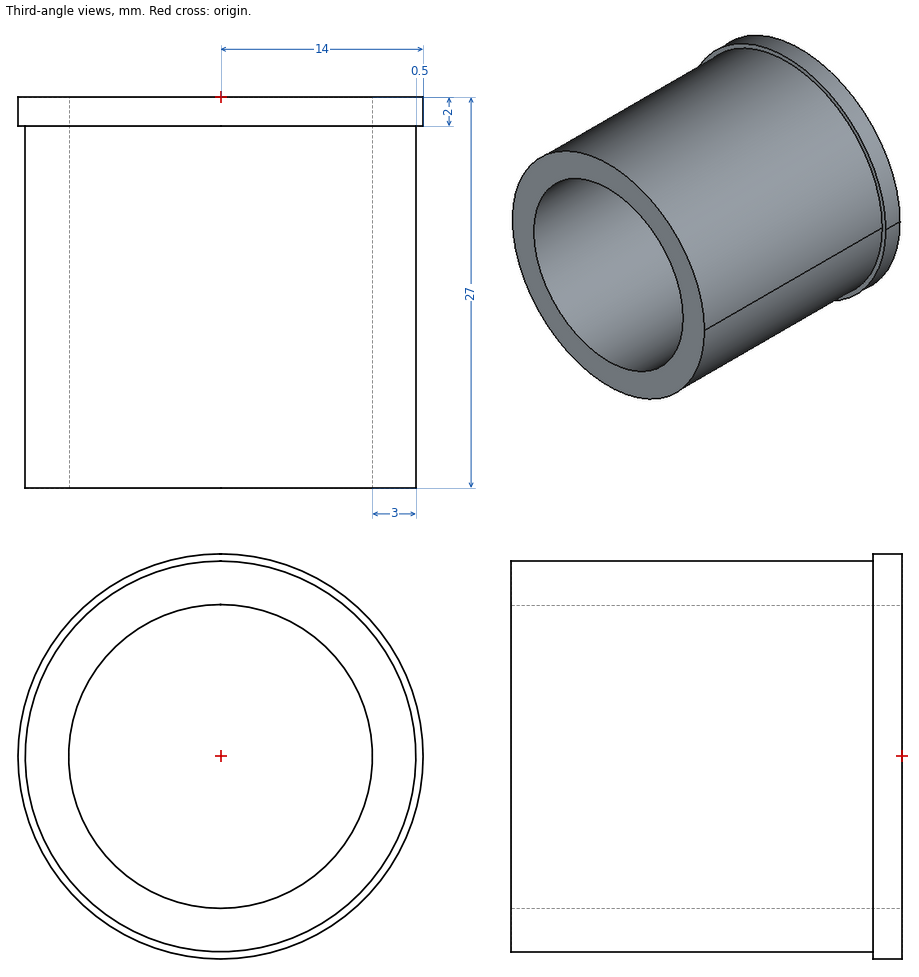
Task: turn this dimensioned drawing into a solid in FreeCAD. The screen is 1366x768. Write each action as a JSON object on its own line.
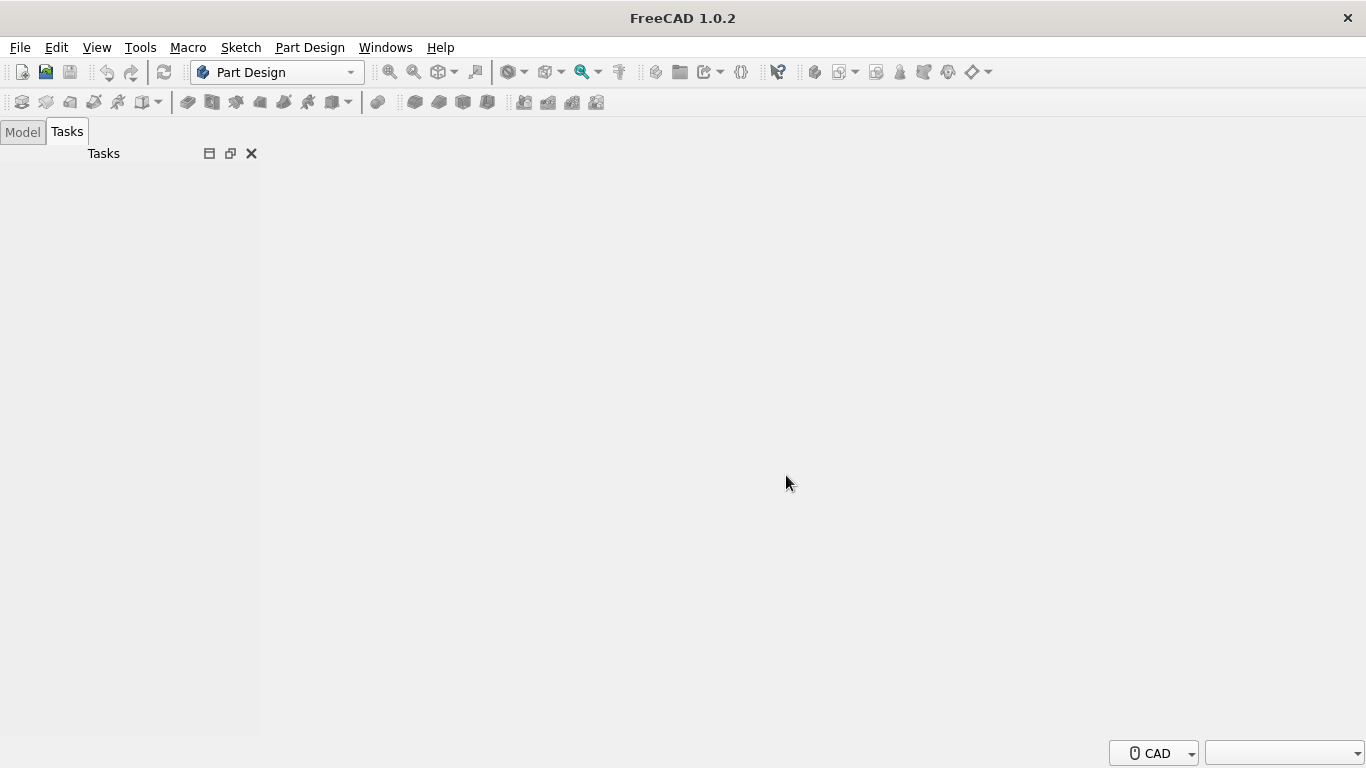
{"action": "key", "text": "ctrl+n"}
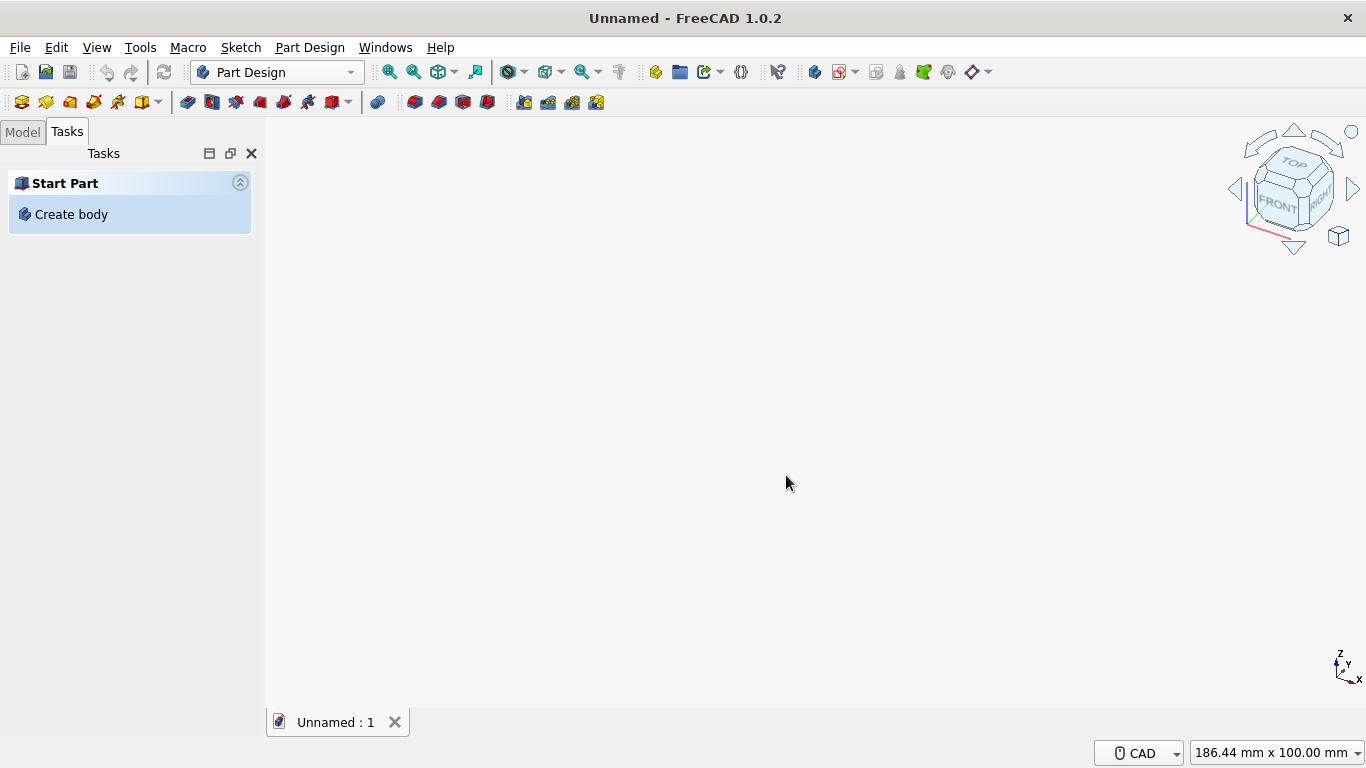
{"action": "left_click", "coordinate": [840, 72]}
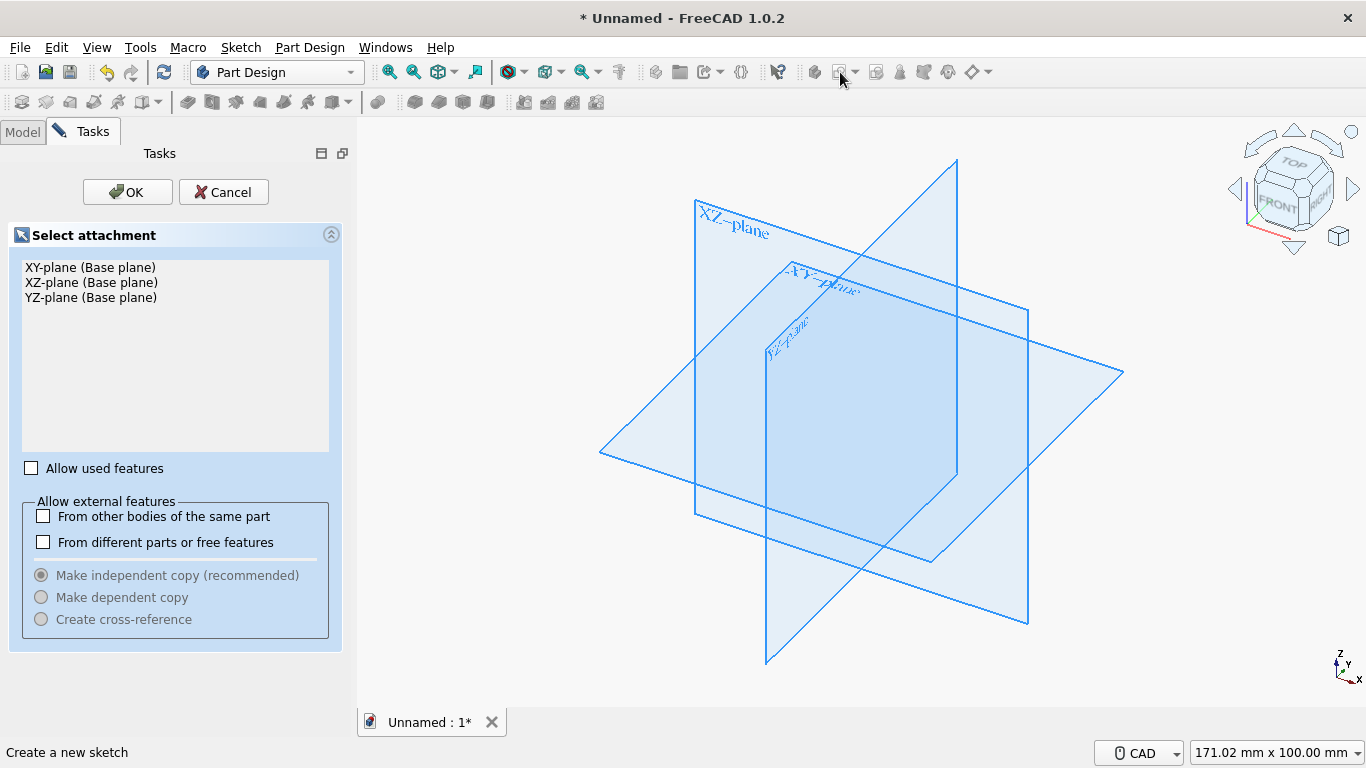
{"action": "left_click", "coordinate": [82, 268]}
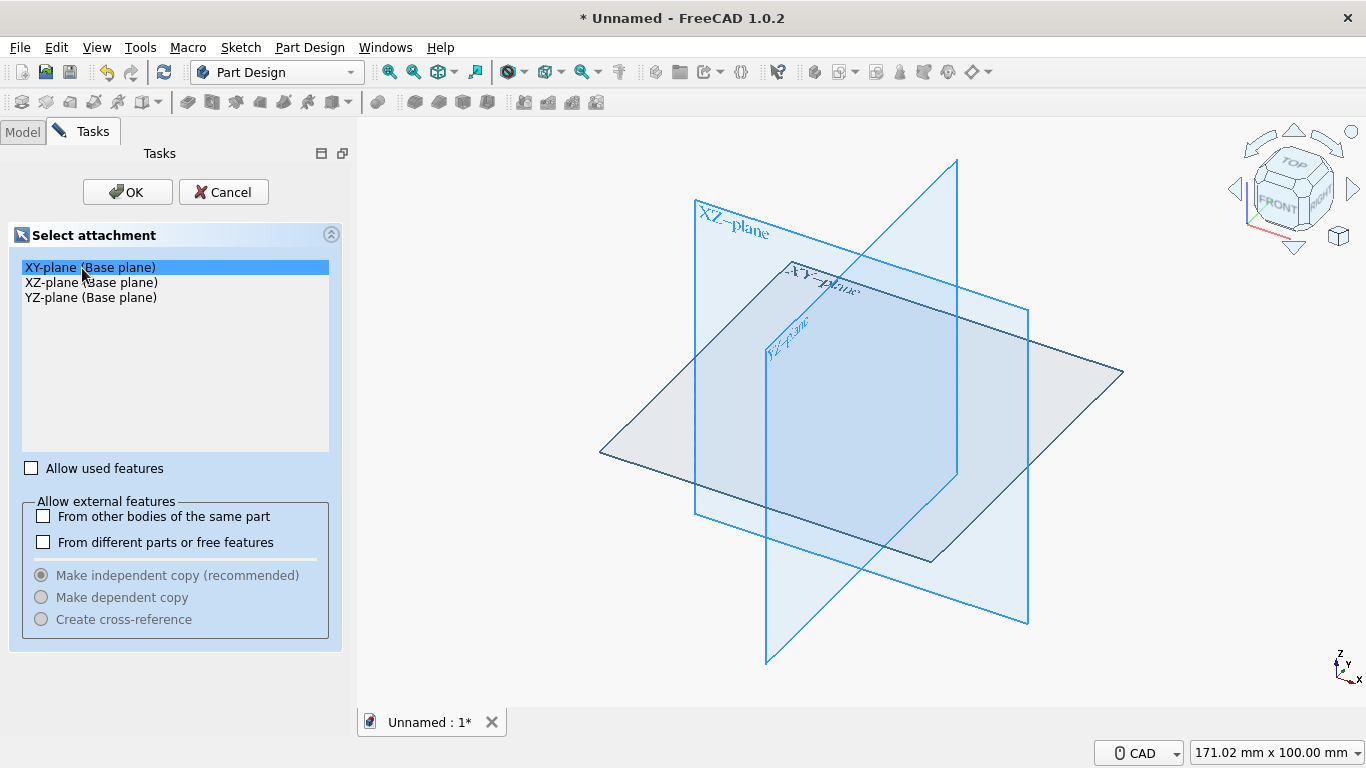
{"action": "left_click", "coordinate": [128, 192]}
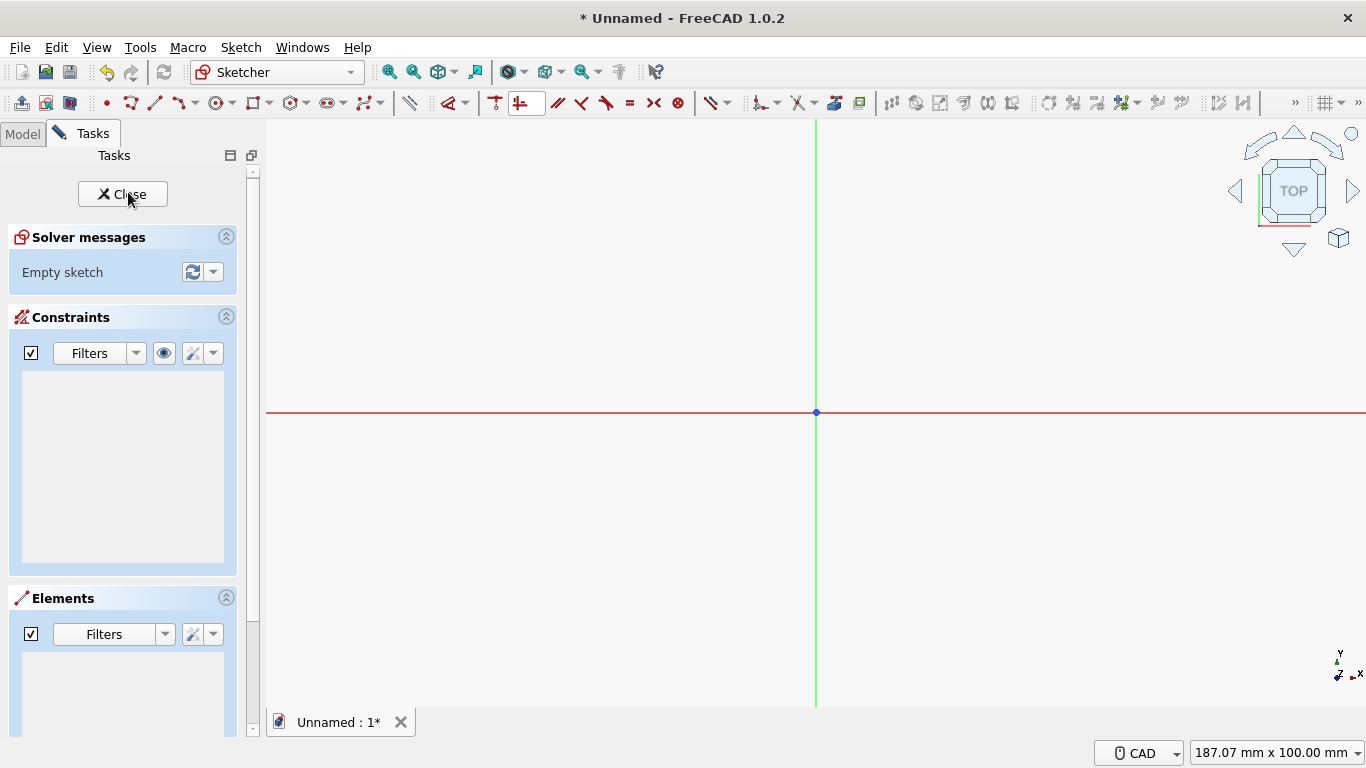
{"action": "scroll", "coordinate": [947, 557], "scroll_direction": "up", "scroll_amount": 4}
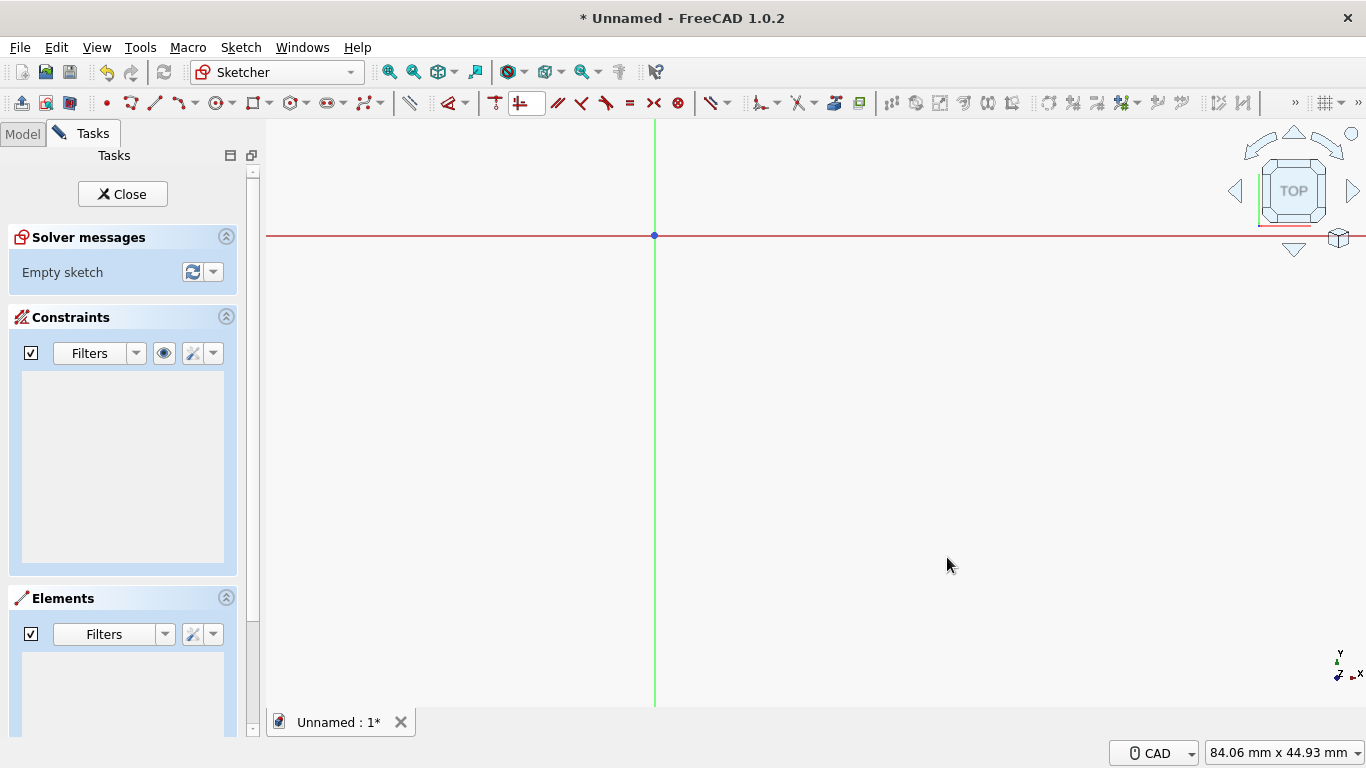
{"action": "key", "text": "g m"}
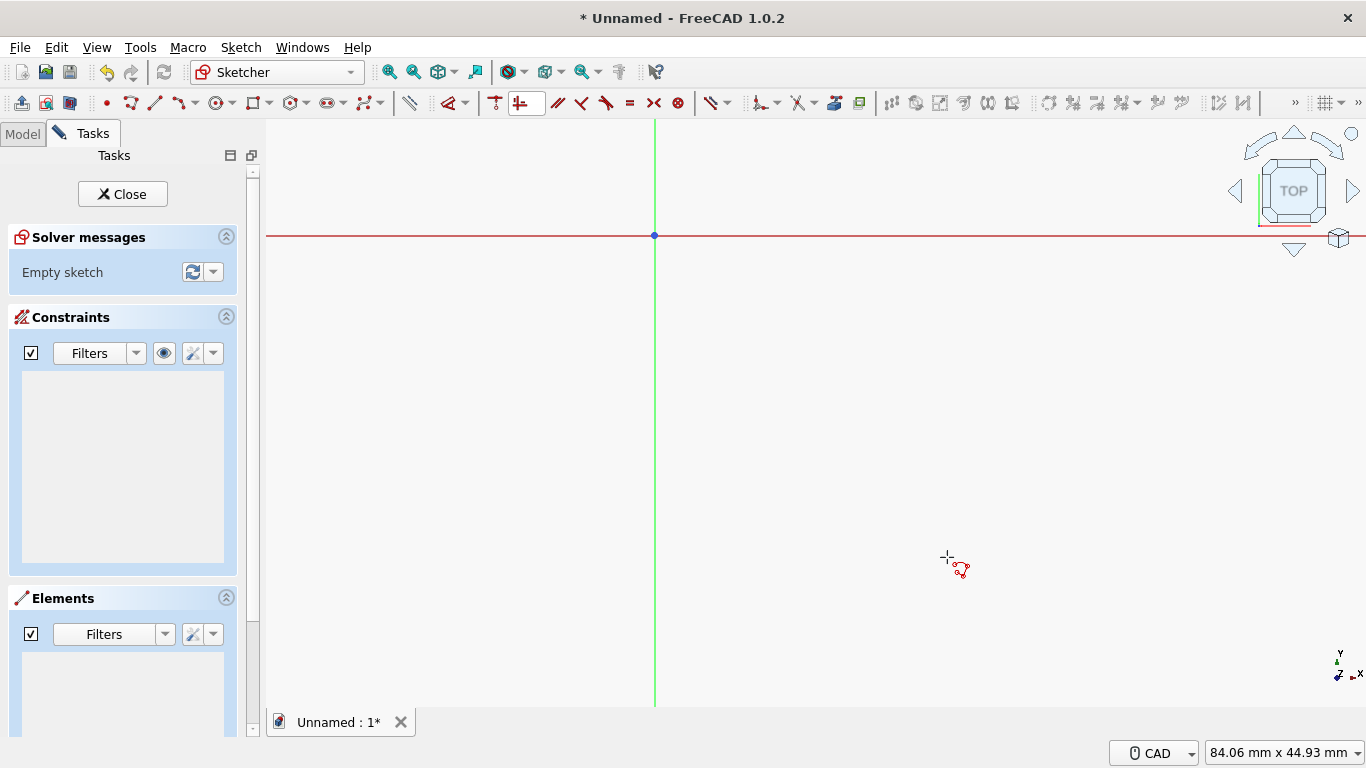
{"action": "left_click", "coordinate": [792, 236]}
{"action": "left_click", "coordinate": [792, 589]}
{"action": "left_click", "coordinate": [831, 589]}
{"action": "left_click", "coordinate": [831, 262]}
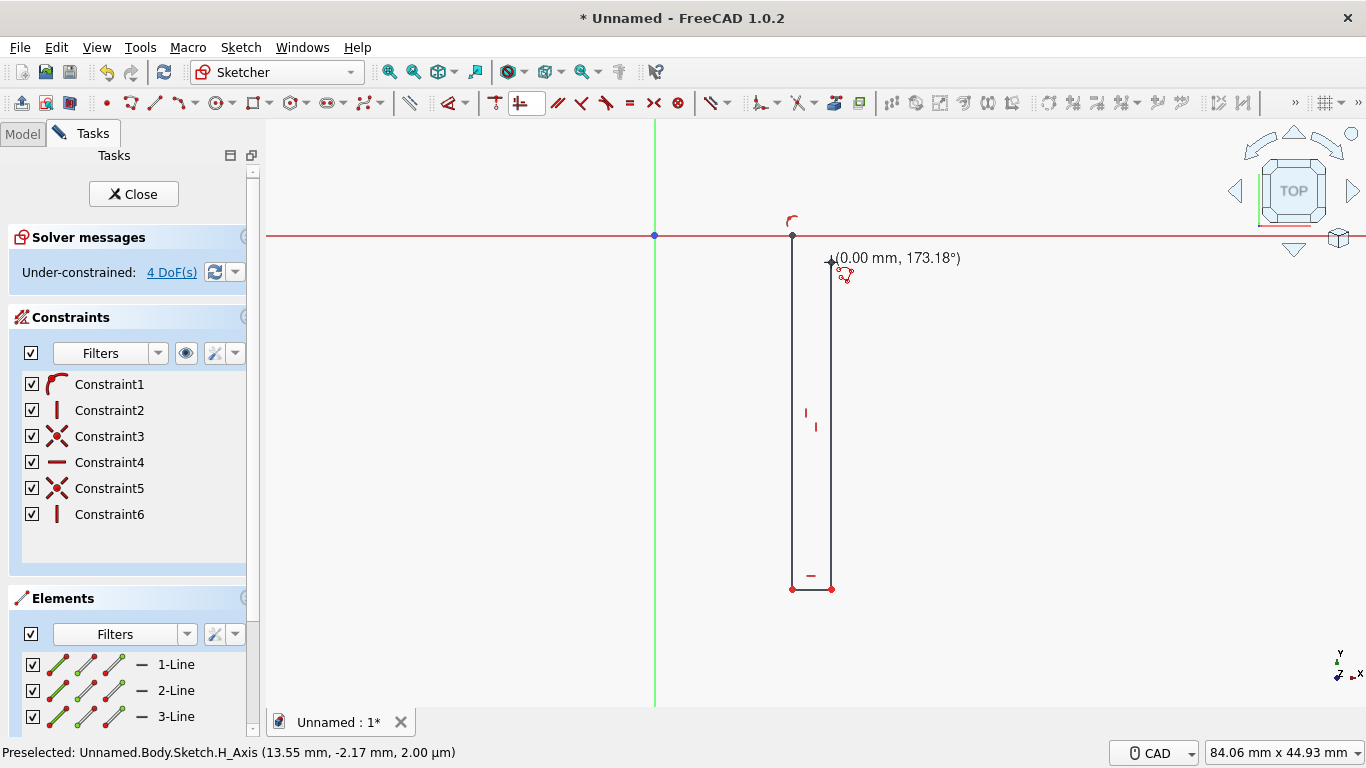
{"action": "scroll", "coordinate": [838, 262], "scroll_direction": "up", "scroll_amount": 5}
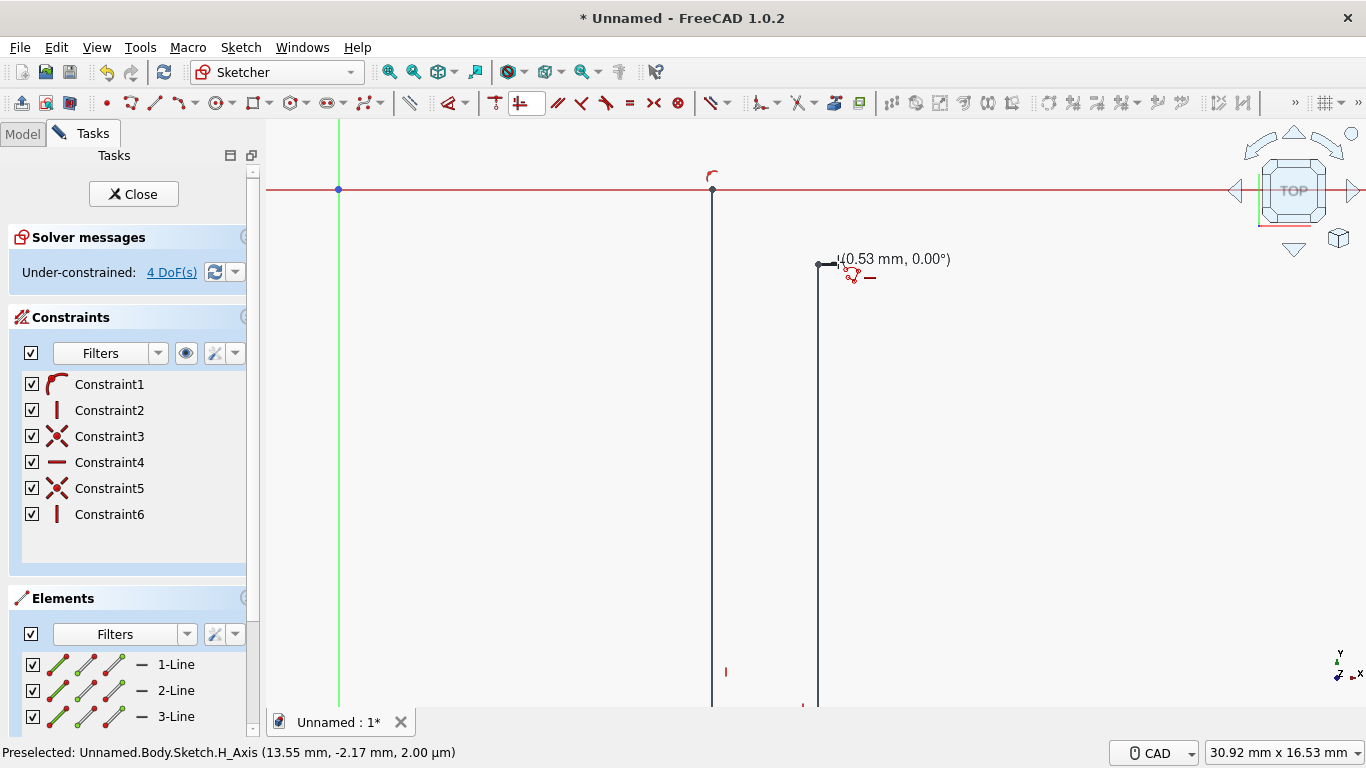
{"action": "left_click", "coordinate": [837, 262]}
{"action": "left_click", "coordinate": [837, 199]}
{"action": "left_click", "coordinate": [712, 190]}
{"action": "key", "text": "Escape"}
{"action": "key", "text": "Escape"}